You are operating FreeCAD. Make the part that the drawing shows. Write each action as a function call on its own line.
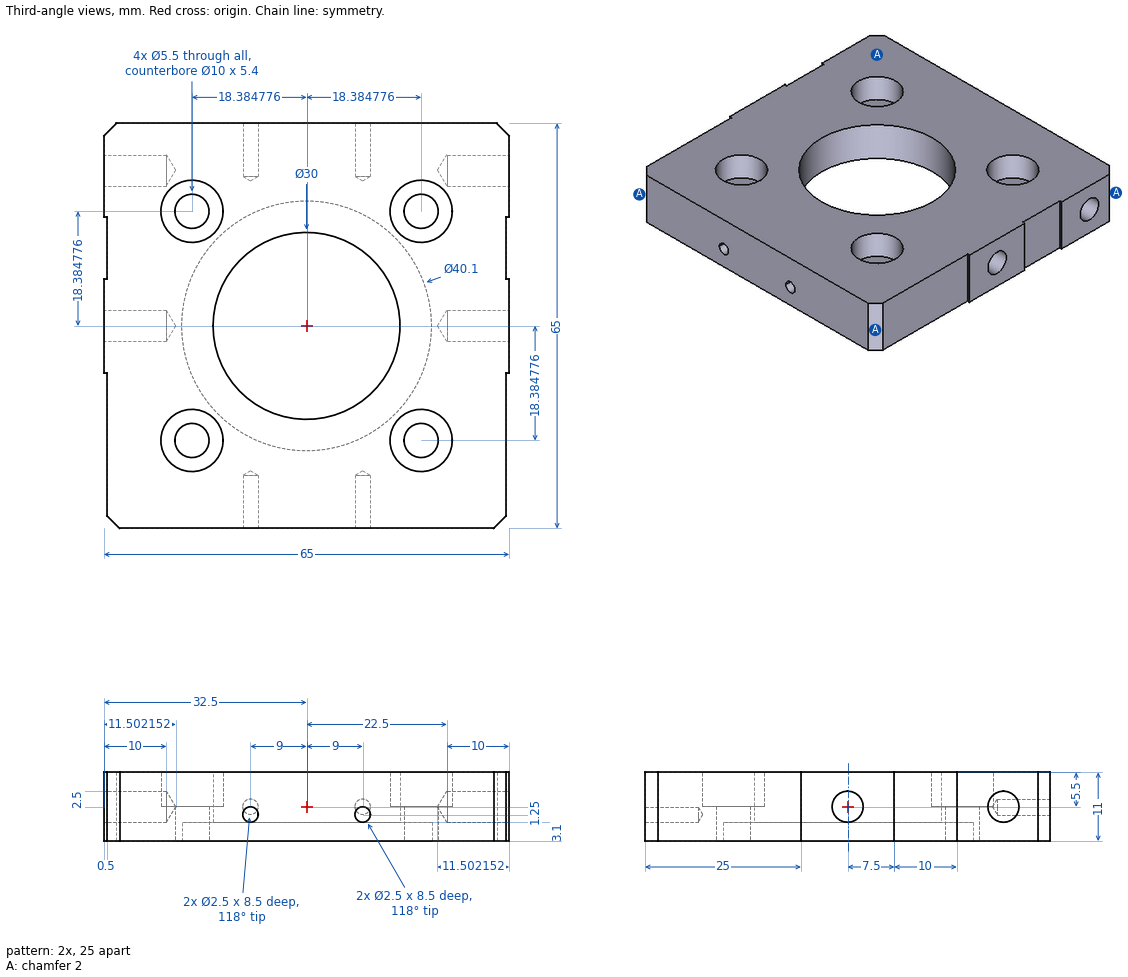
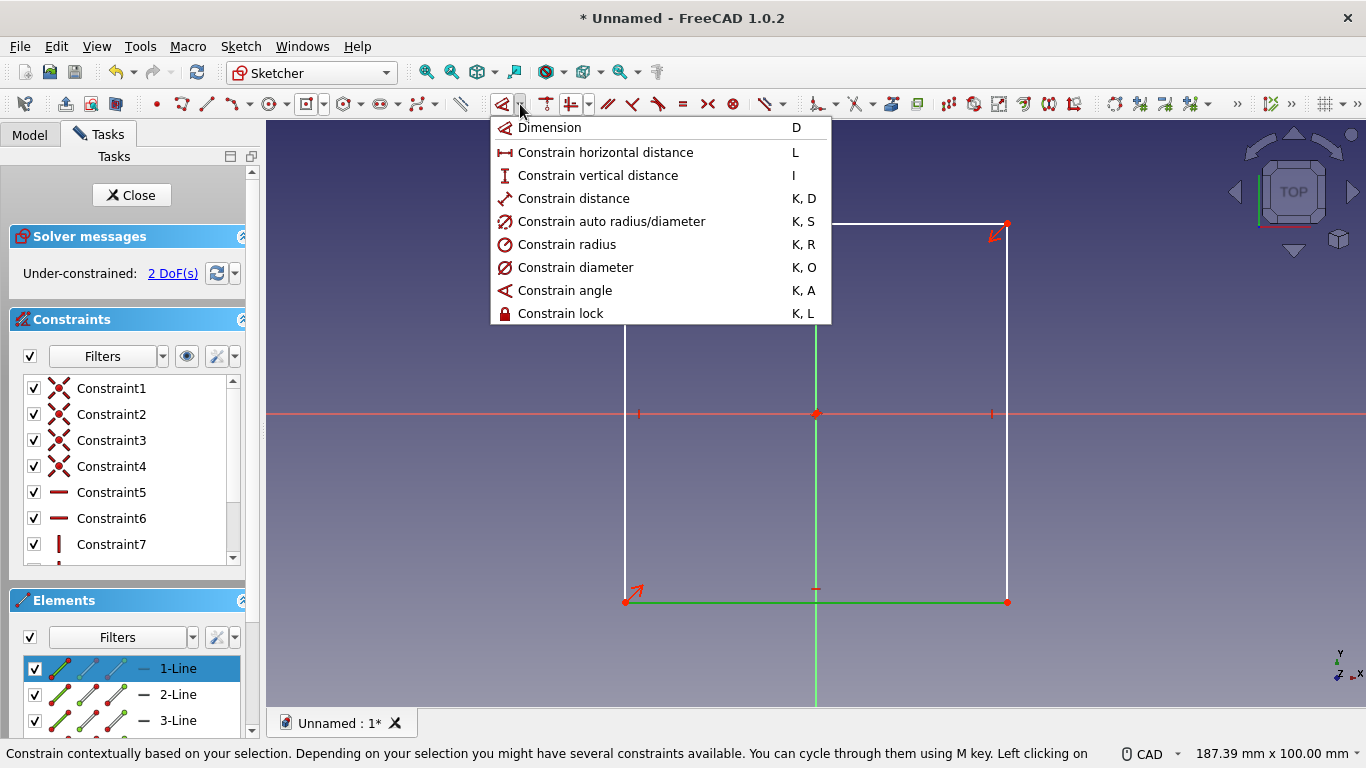
click(661, 152)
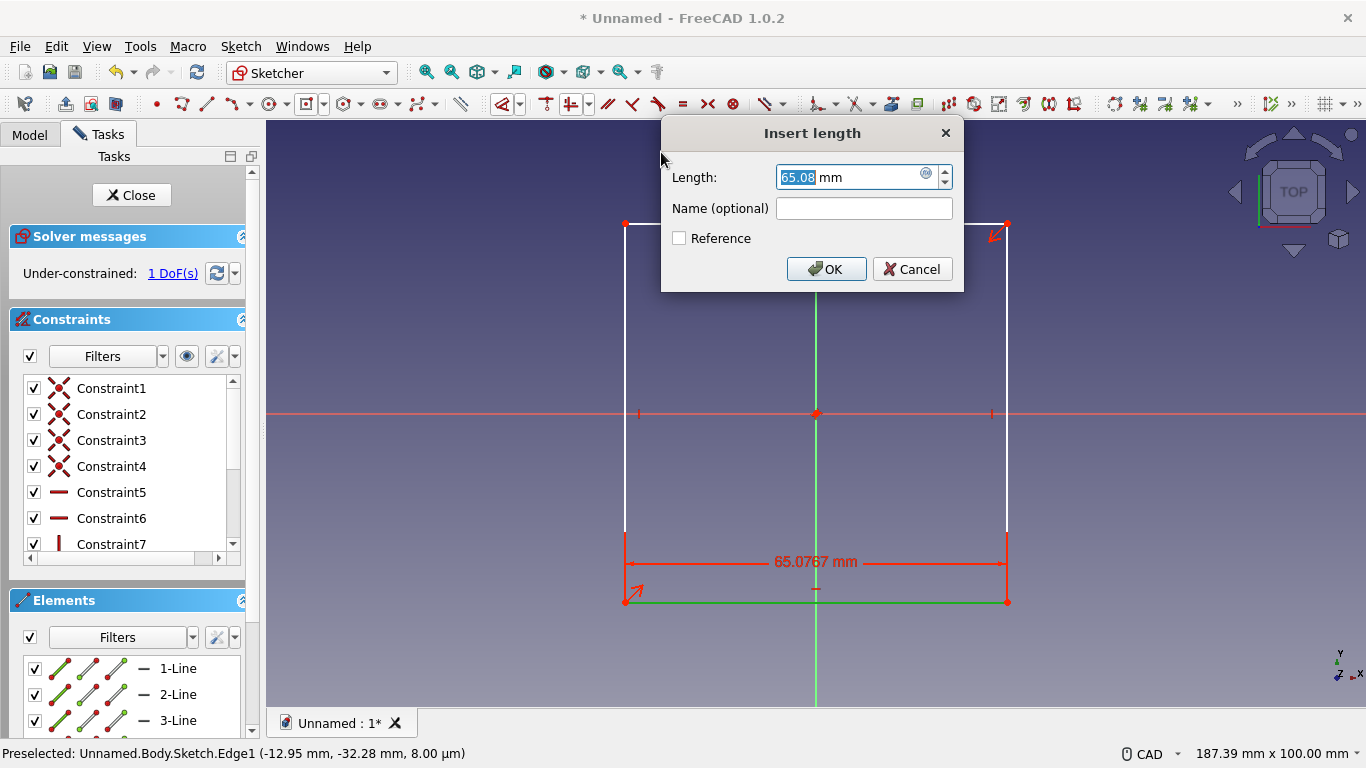
text(65)
key(Return)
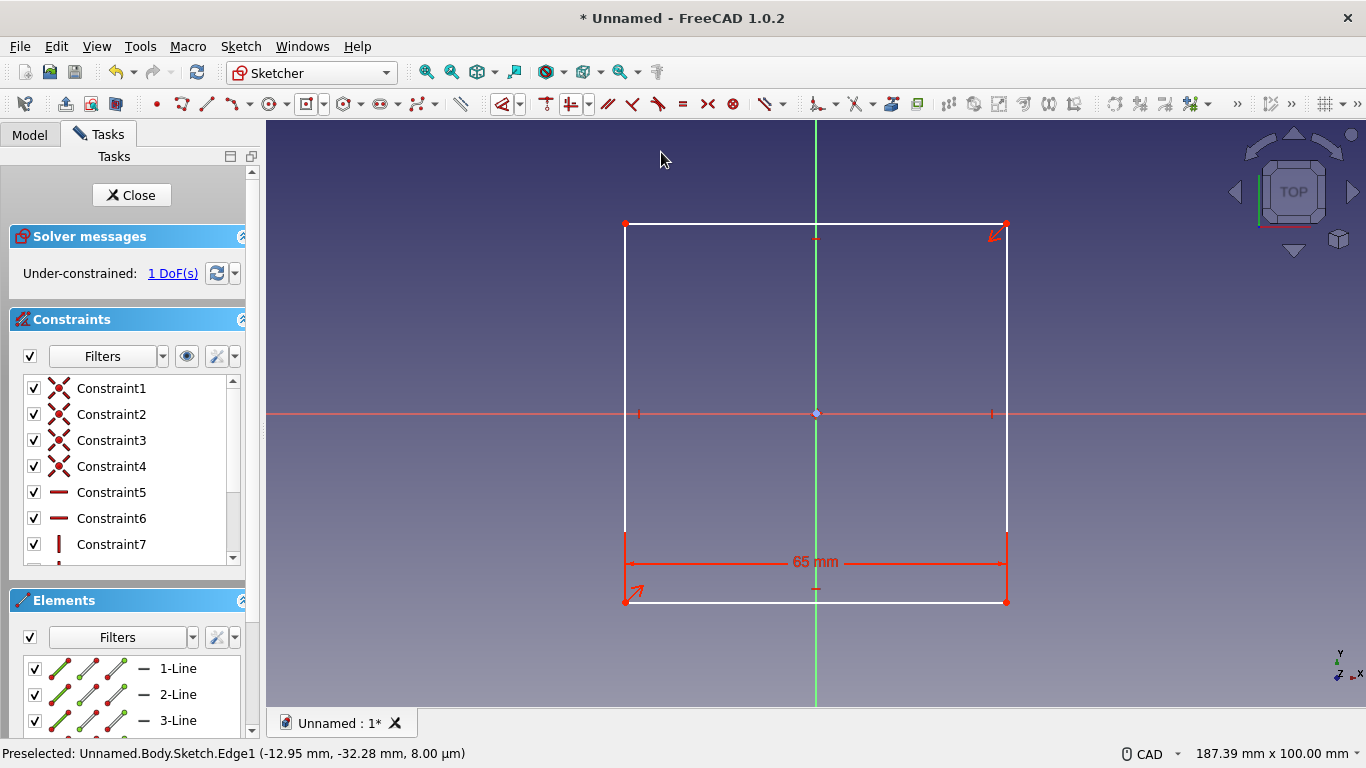
click(1007, 489)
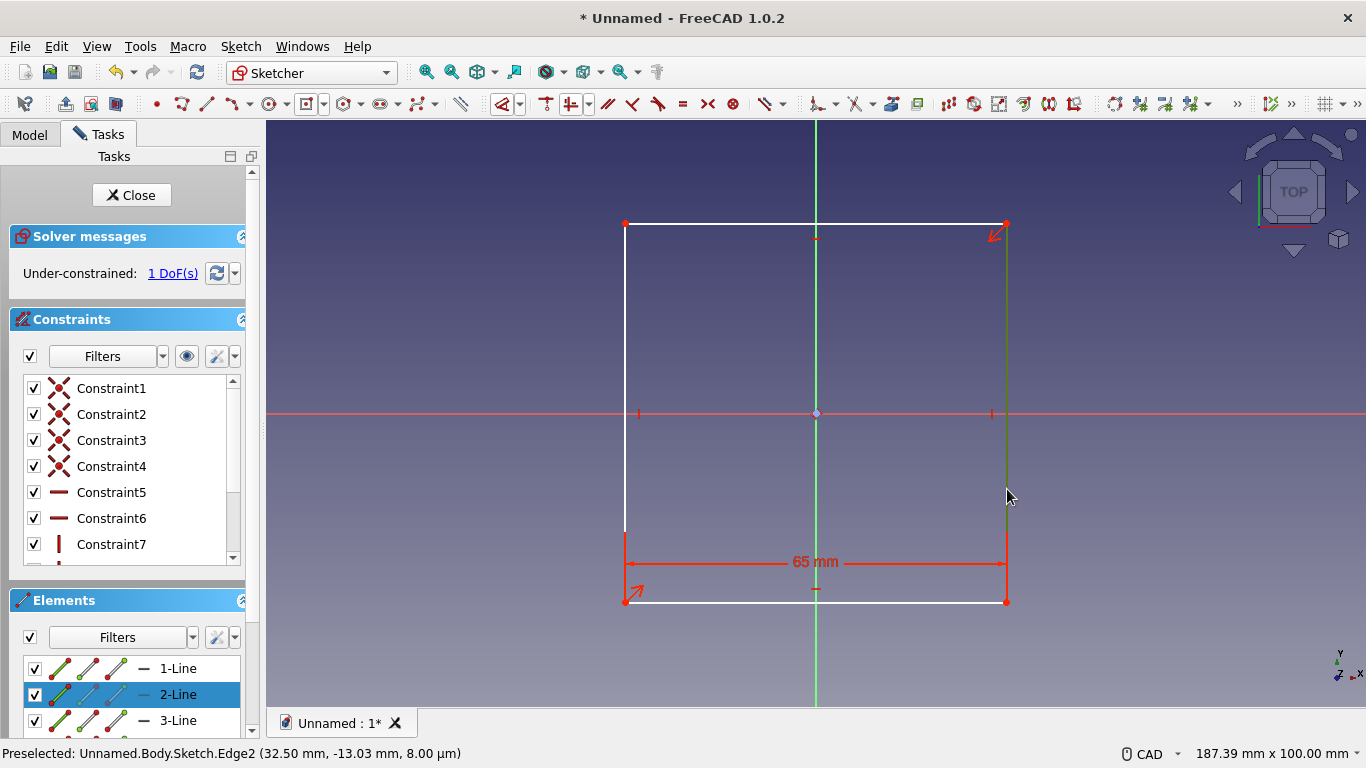
click(520, 104)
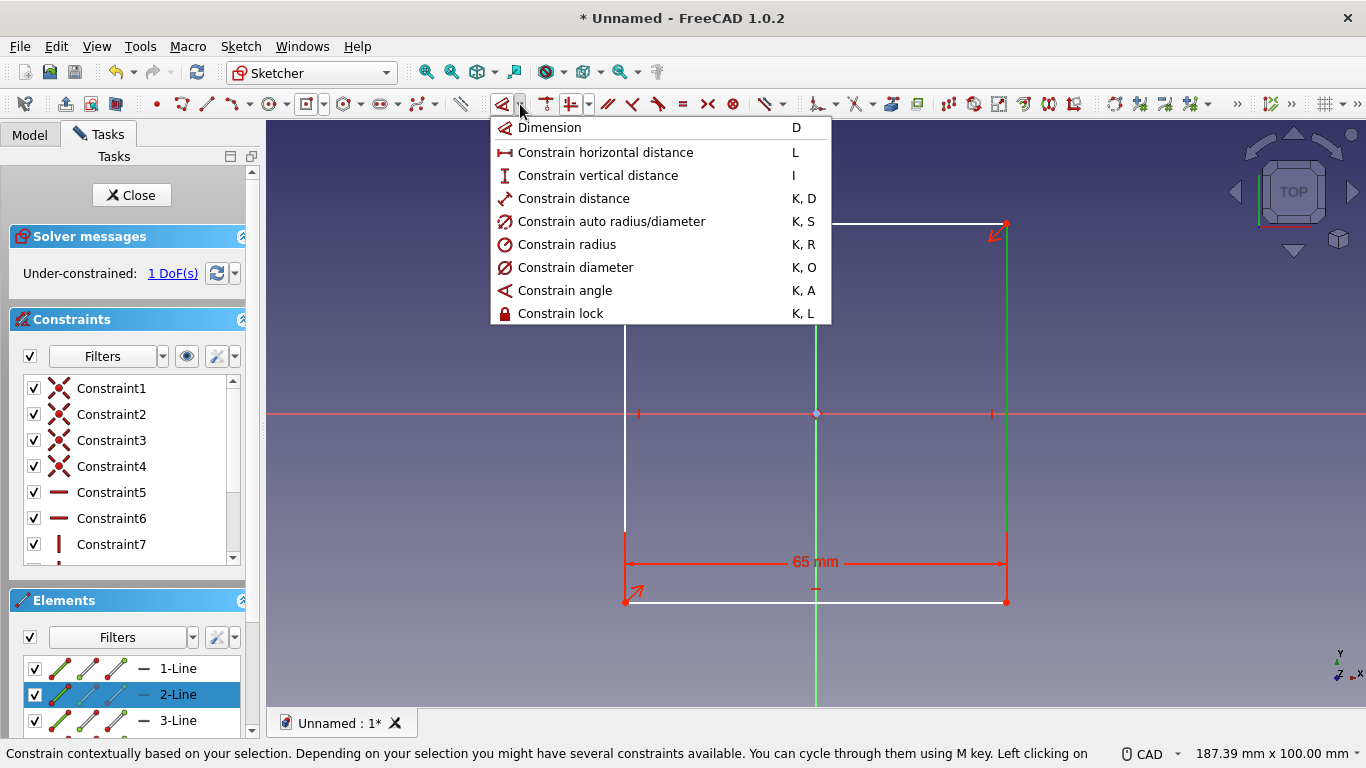
click(661, 176)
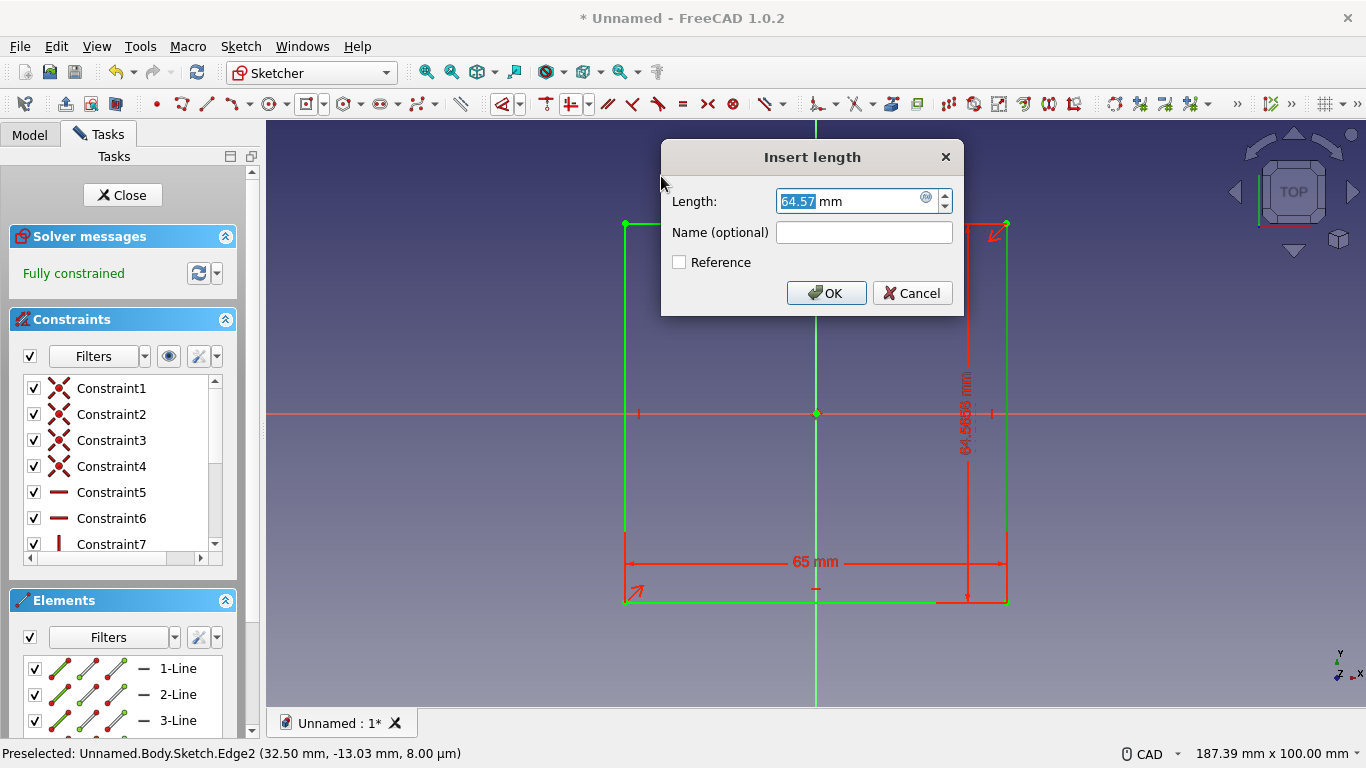
text(65)
key(Return)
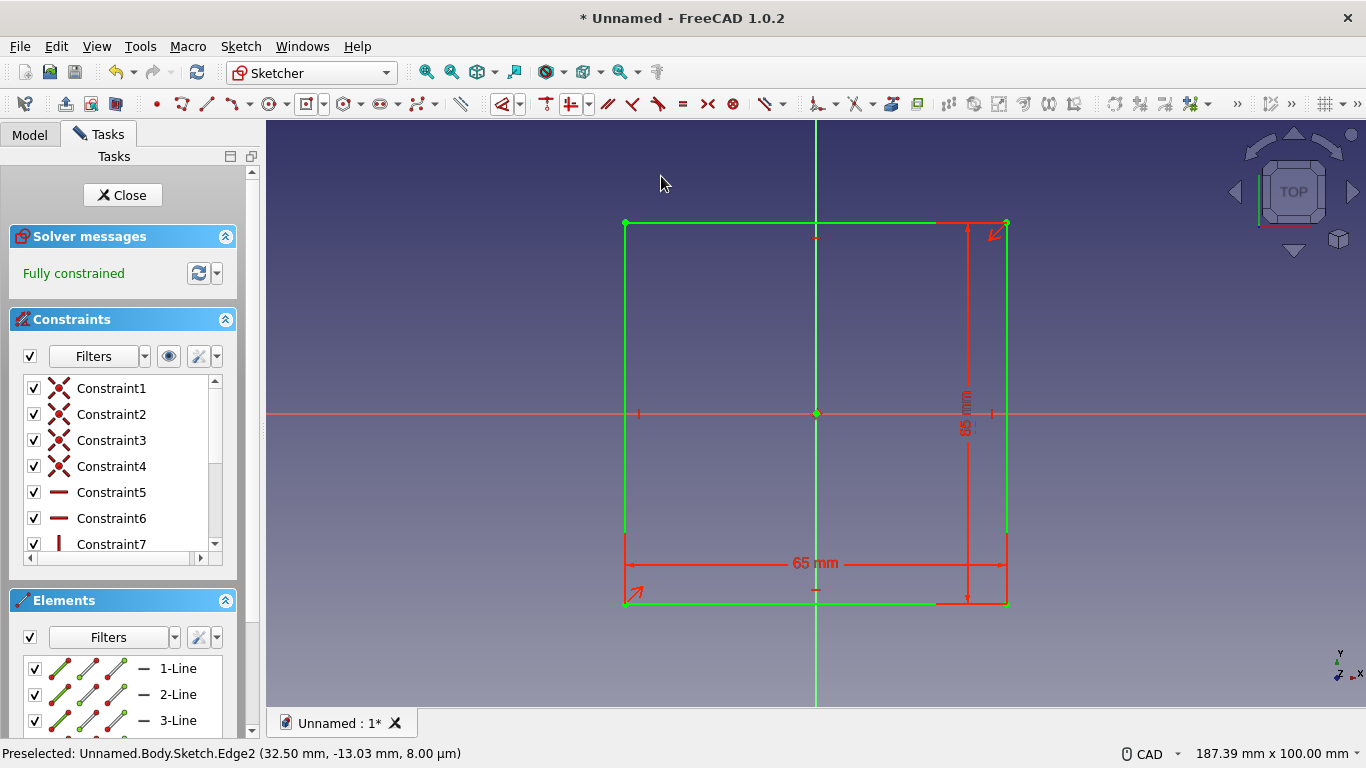
click(123, 195)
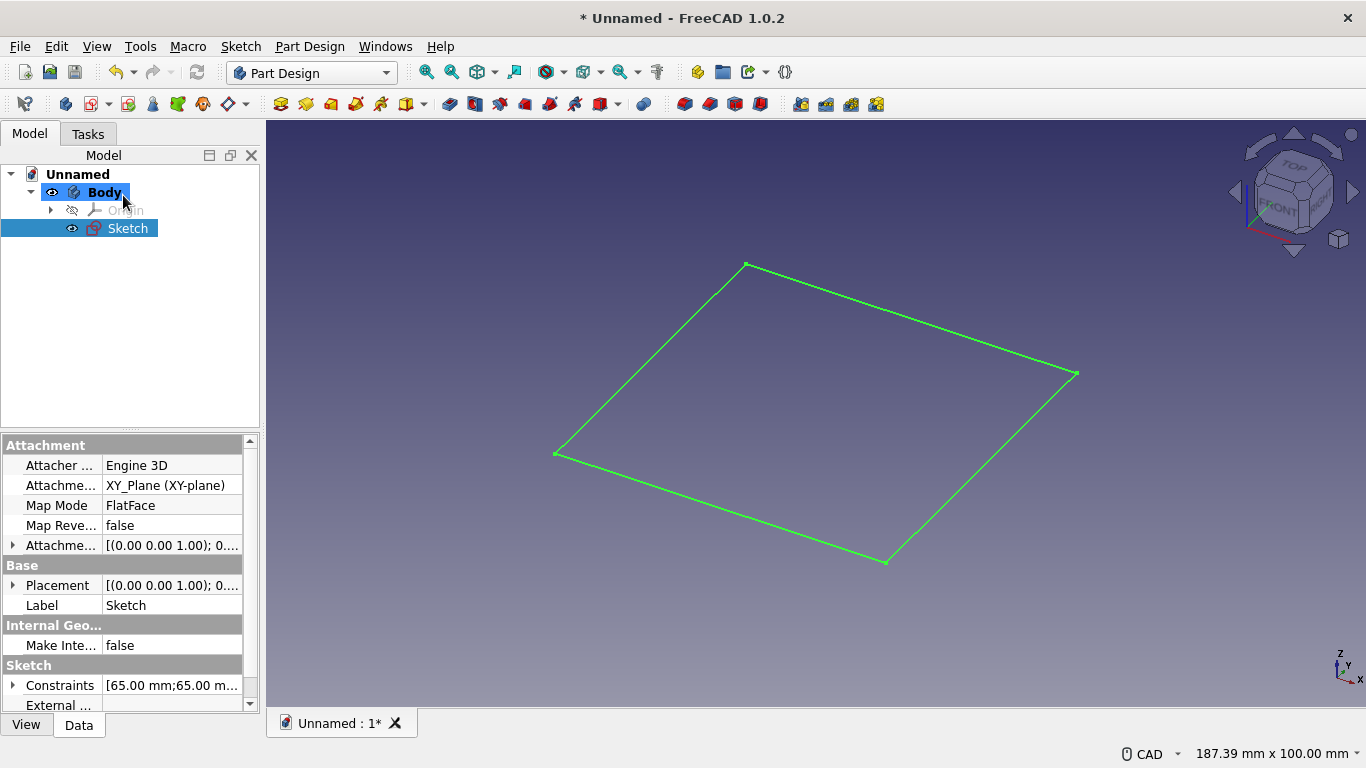
click(281, 104)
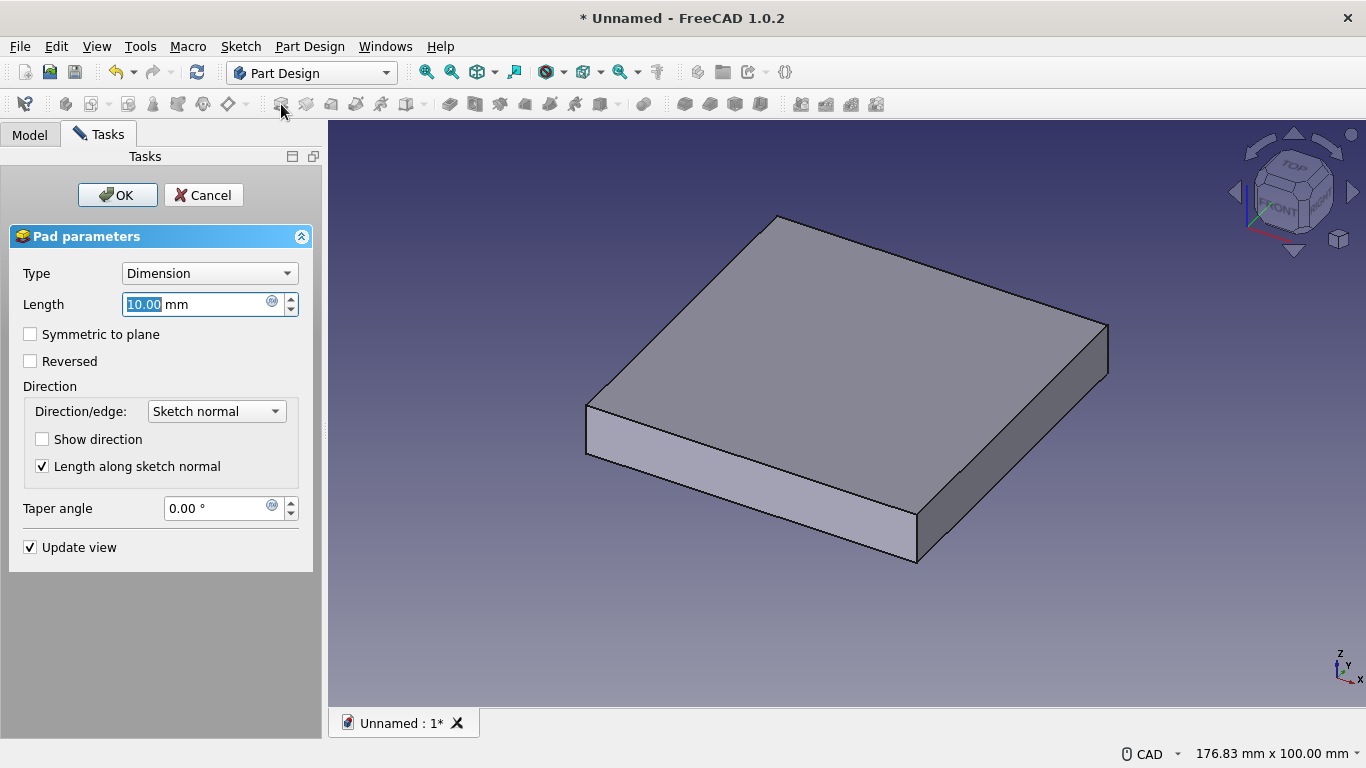
text(11)
key(Tab)